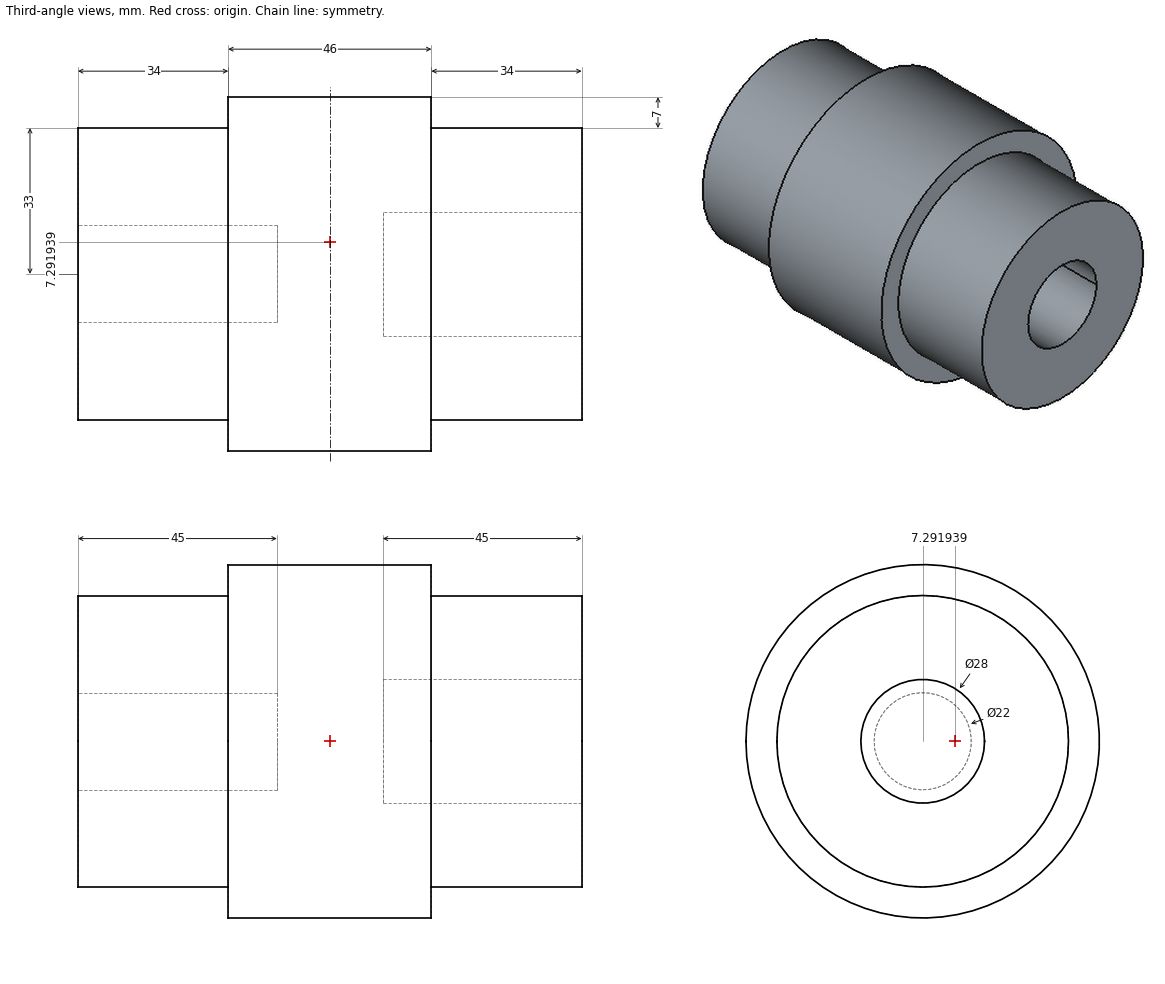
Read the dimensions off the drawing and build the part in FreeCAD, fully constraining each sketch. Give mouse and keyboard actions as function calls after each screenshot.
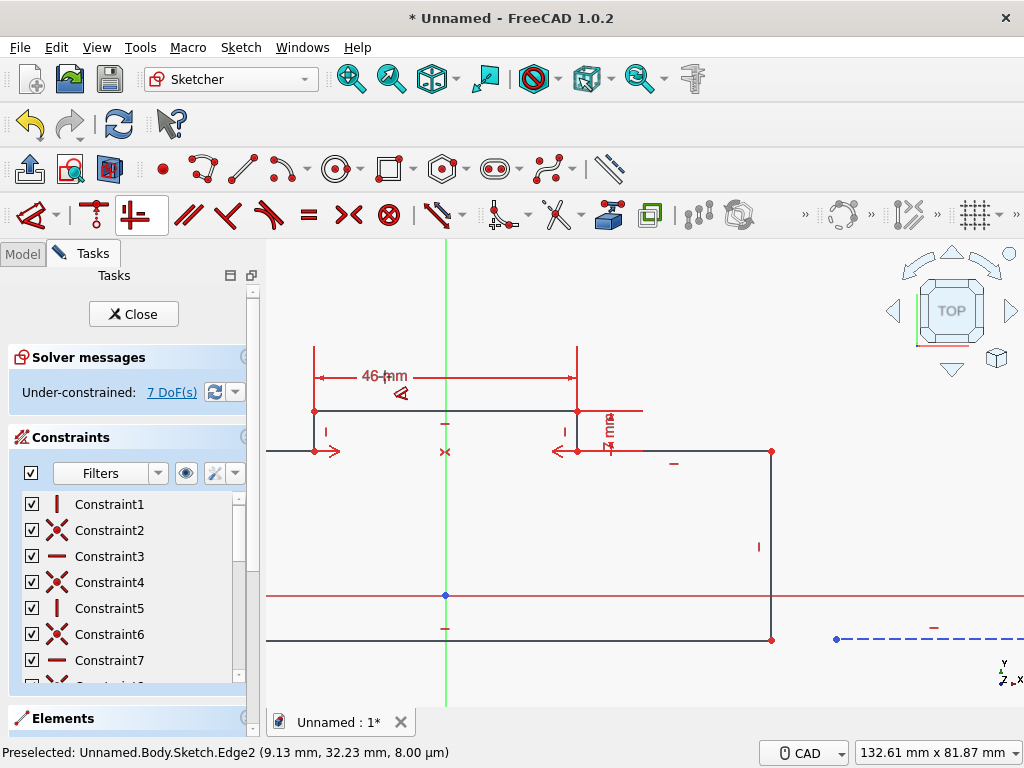
scroll(577, 432, down, 4)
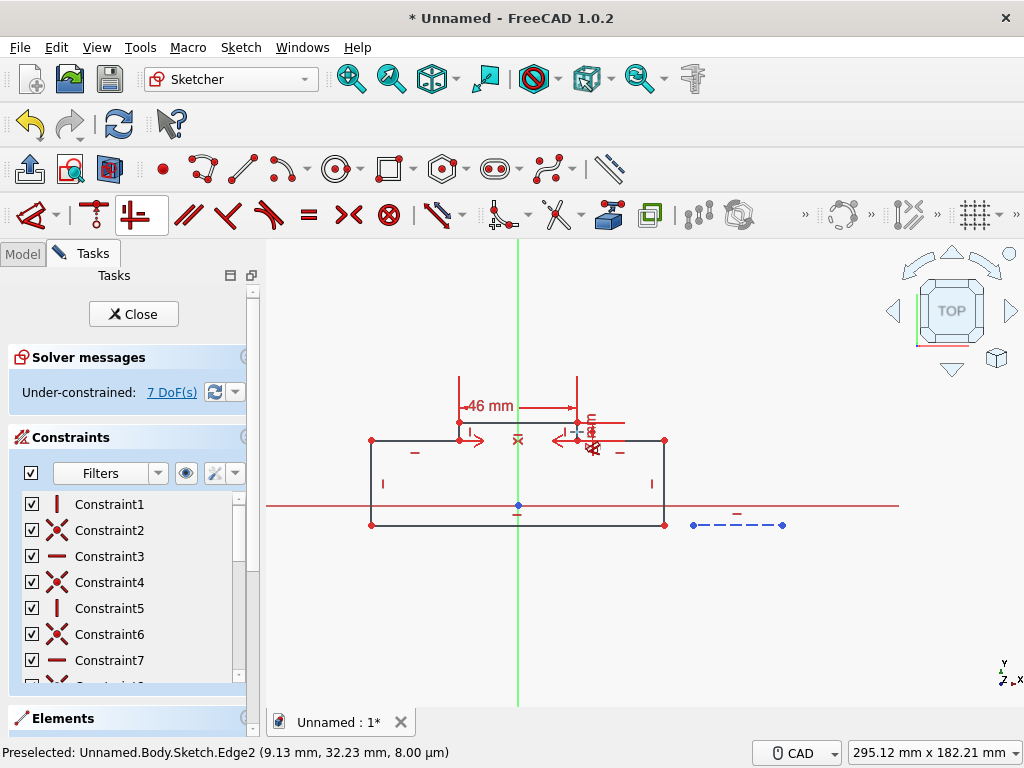
click(433, 441)
click(415, 407)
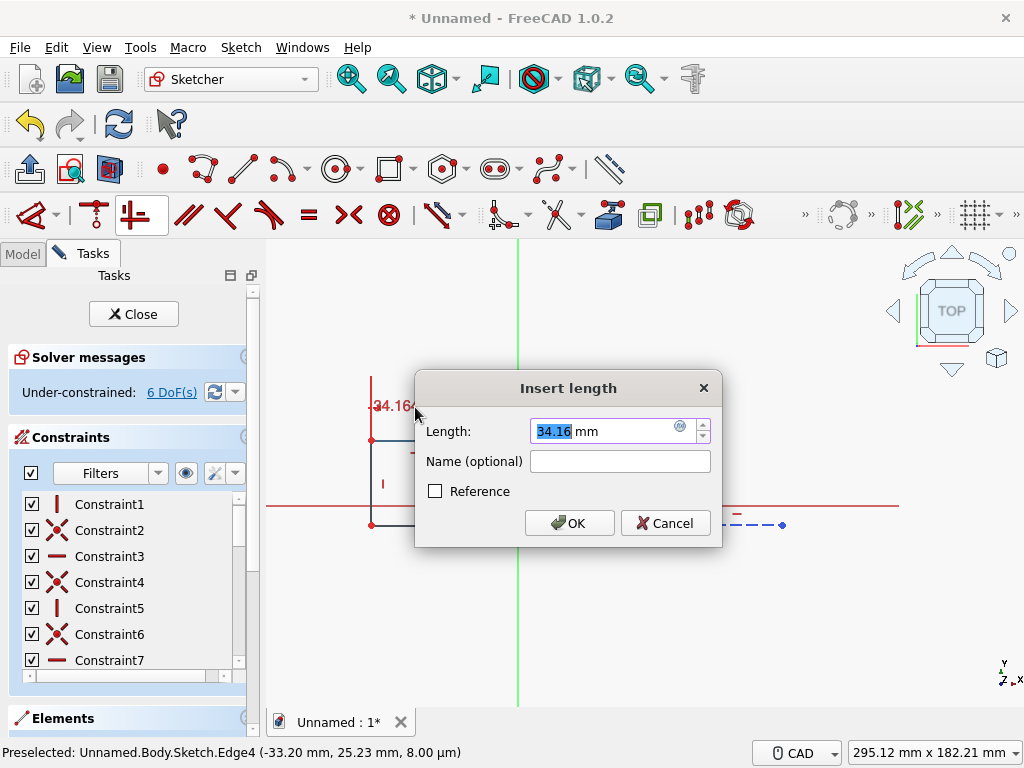
text(34)
key(Return)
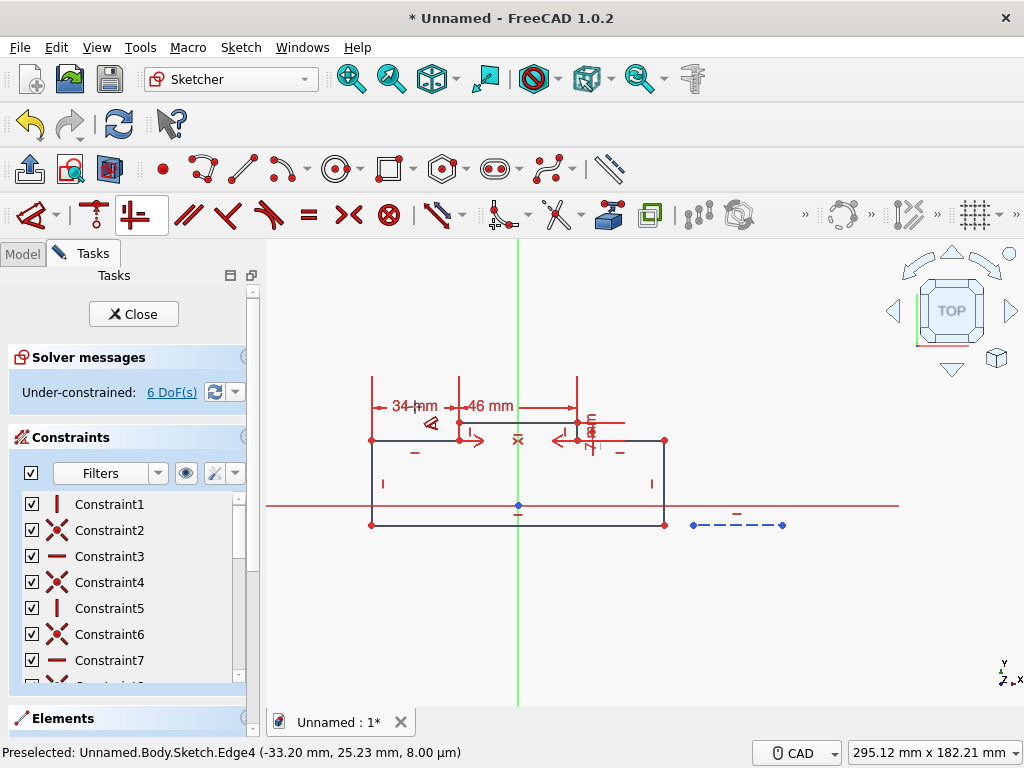
click(372, 466)
click(338, 483)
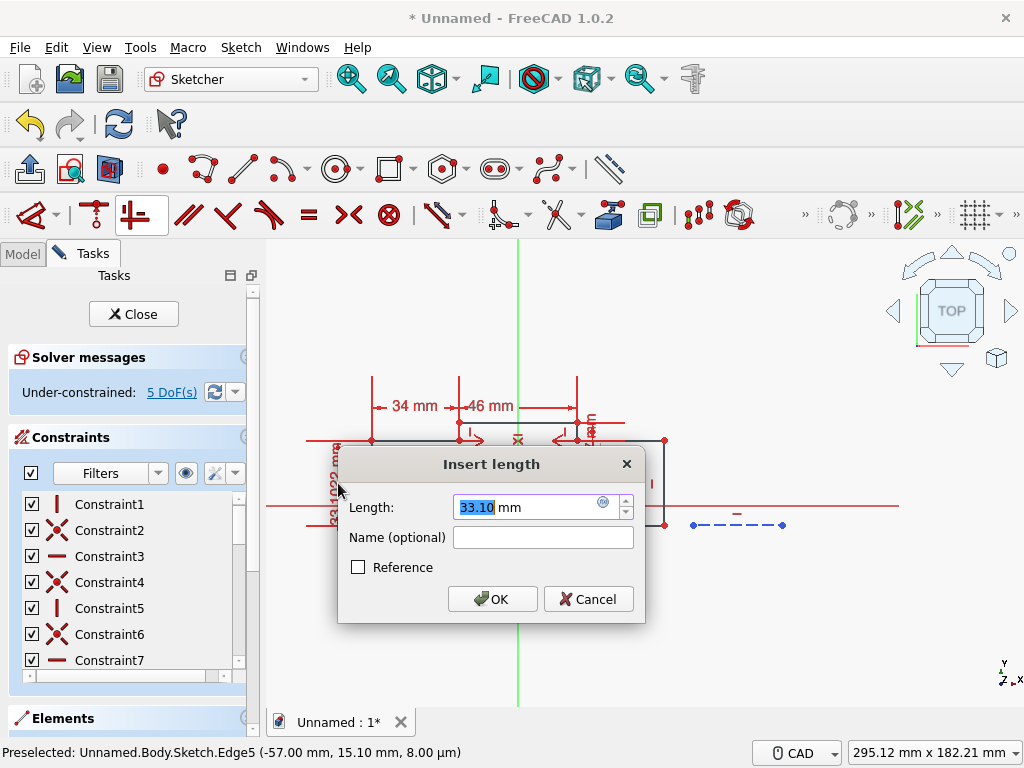
text(33)
key(Return)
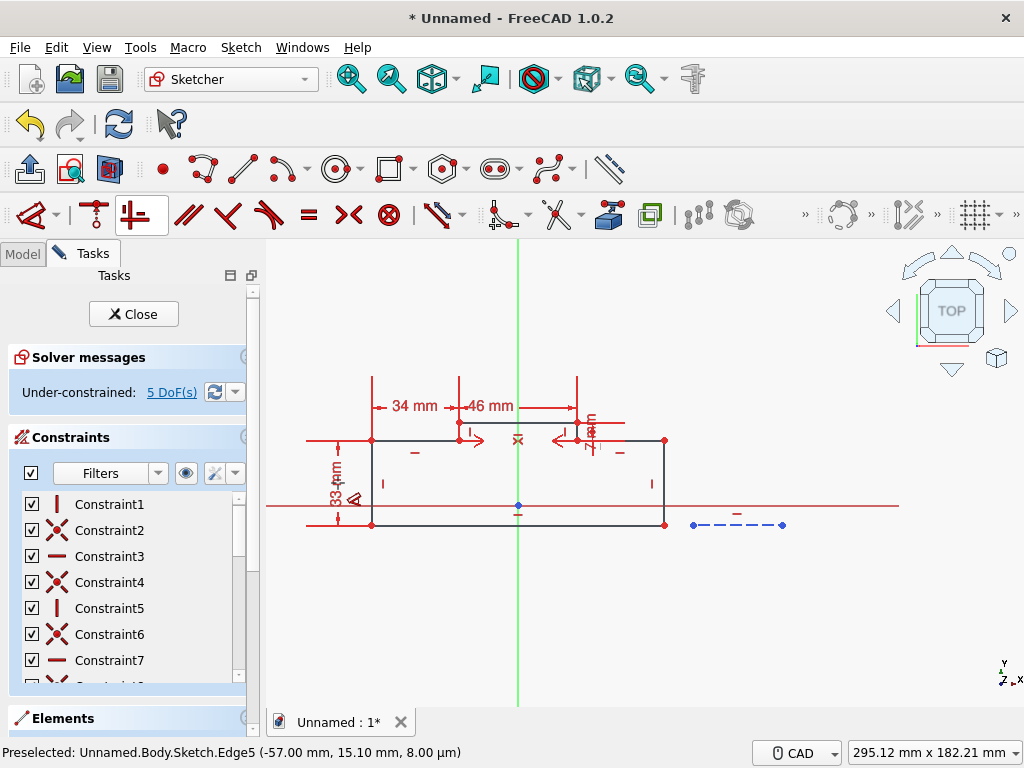
click(638, 441)
click(621, 407)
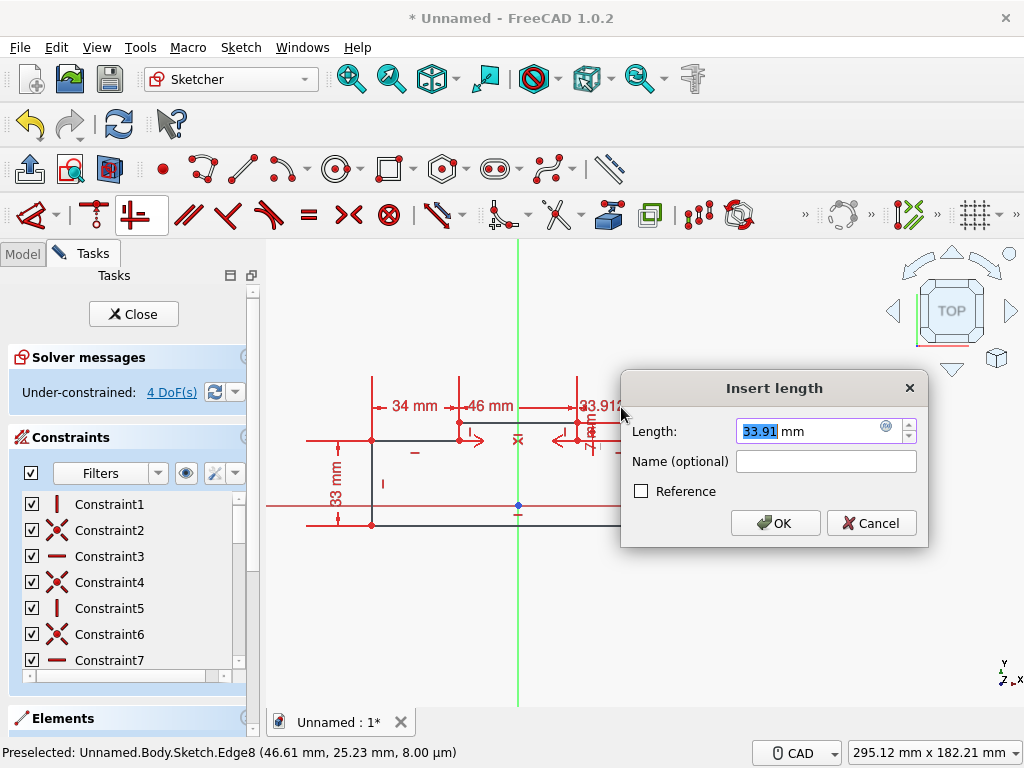
text(34)
key(Return)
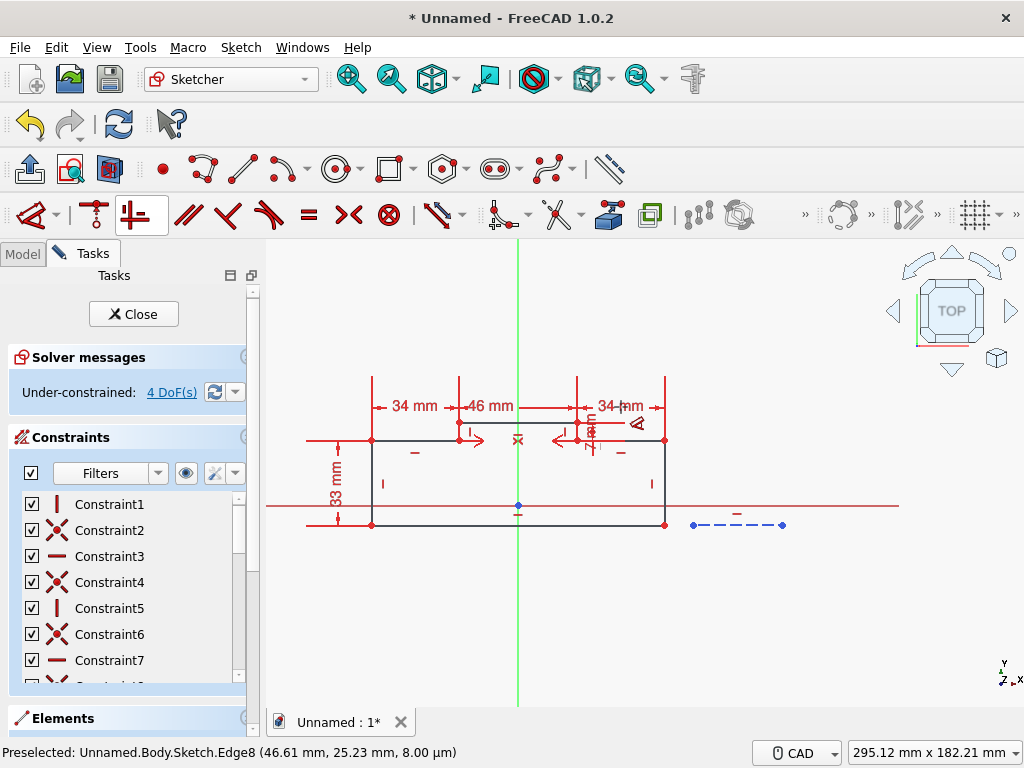
scroll(372, 526, up, 4)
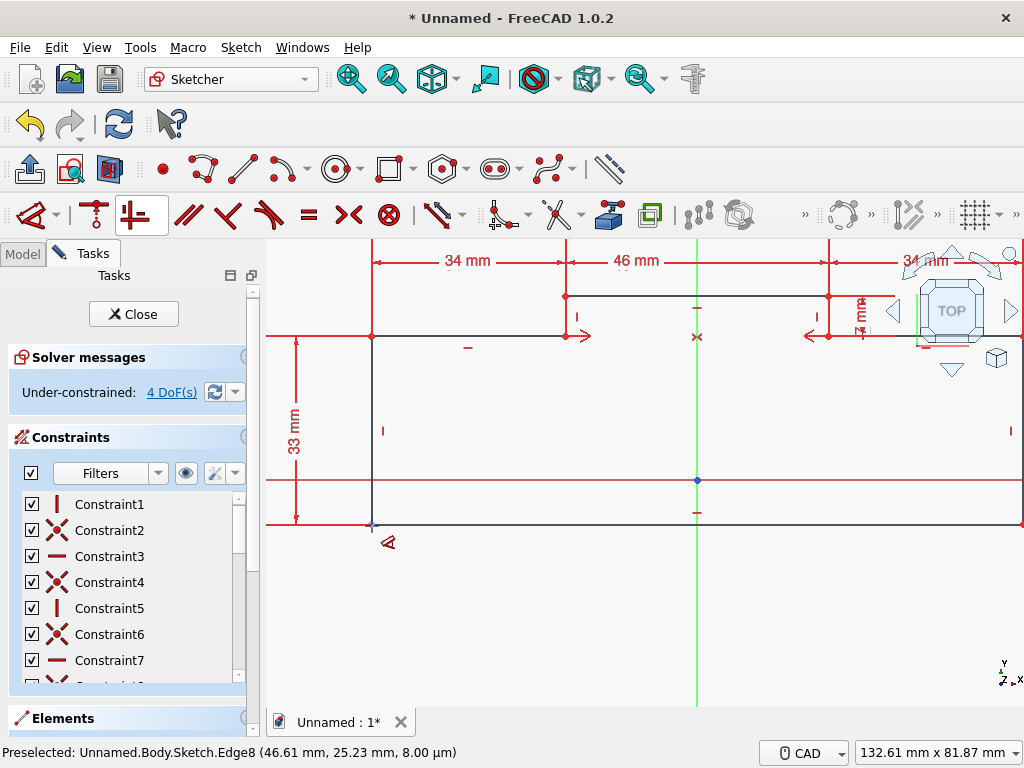
click(372, 525)
click(338, 502)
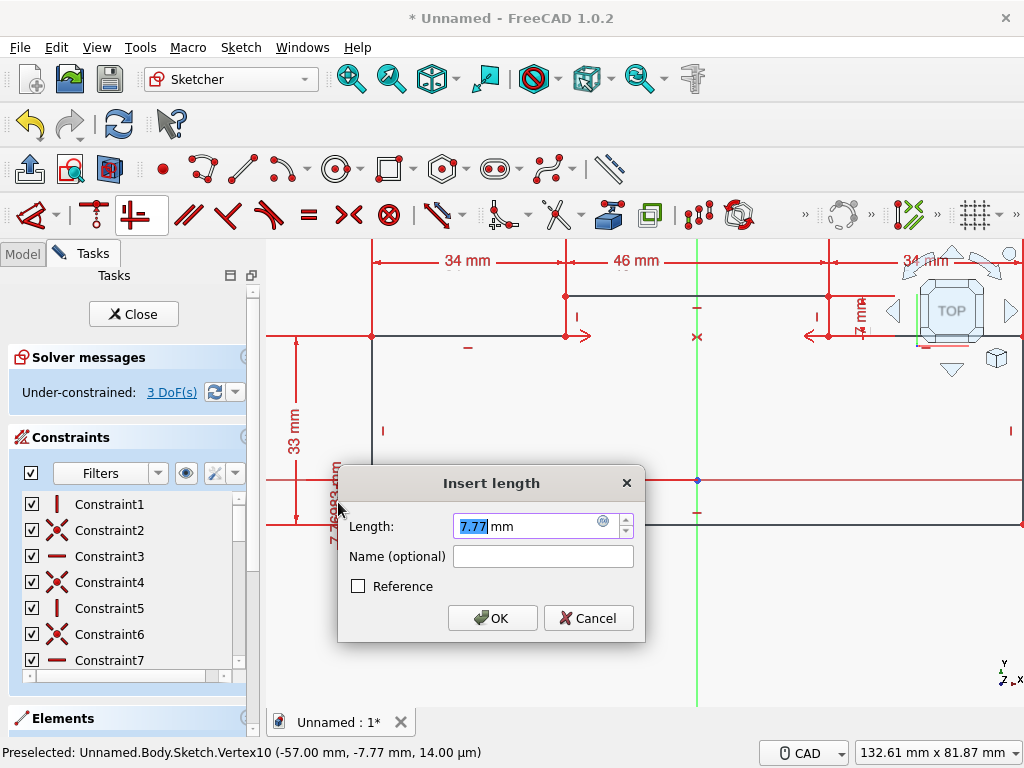
text(7.291939)
key(Return)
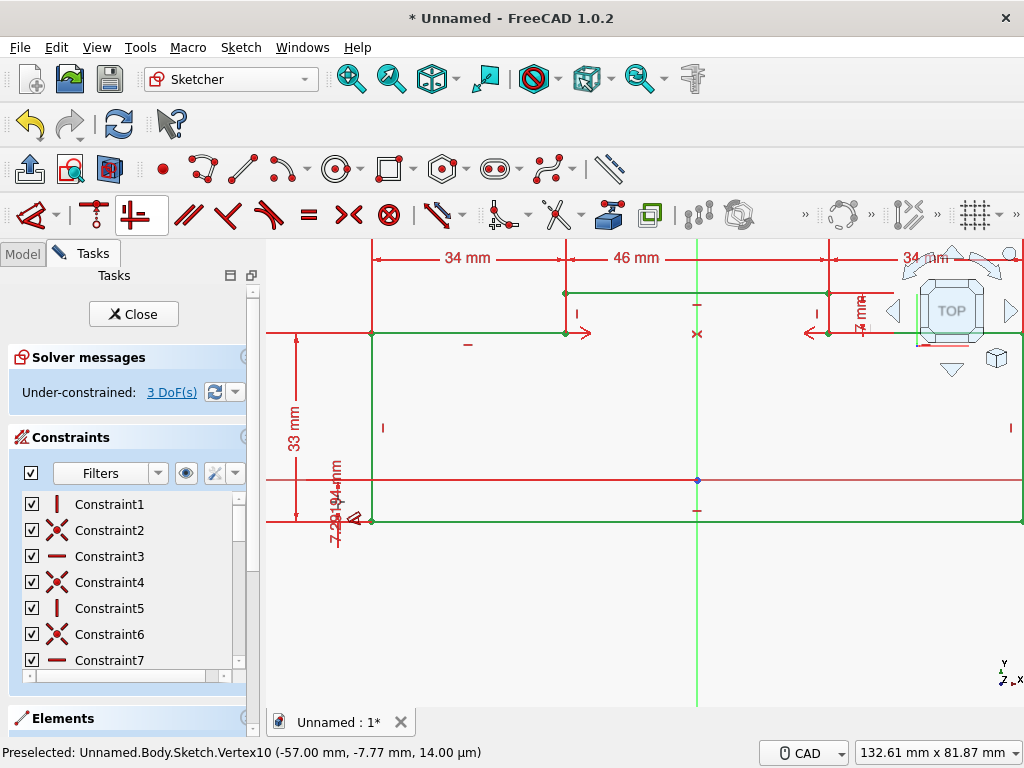
scroll(372, 526, down, 4)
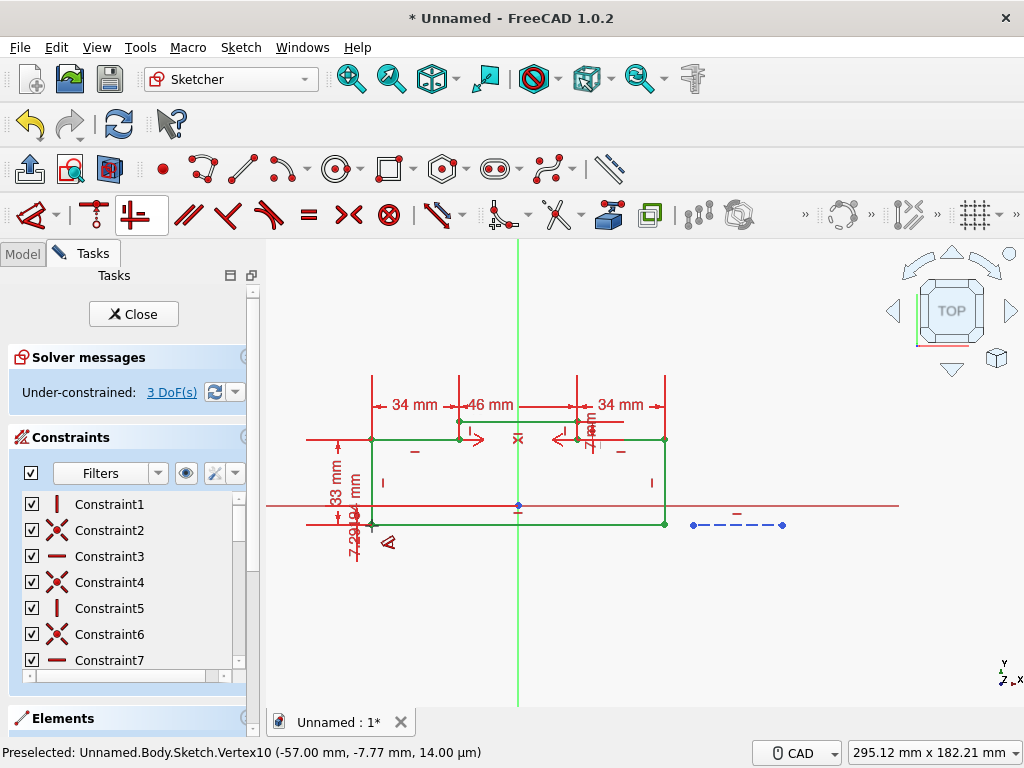
scroll(694, 525, up, 4)